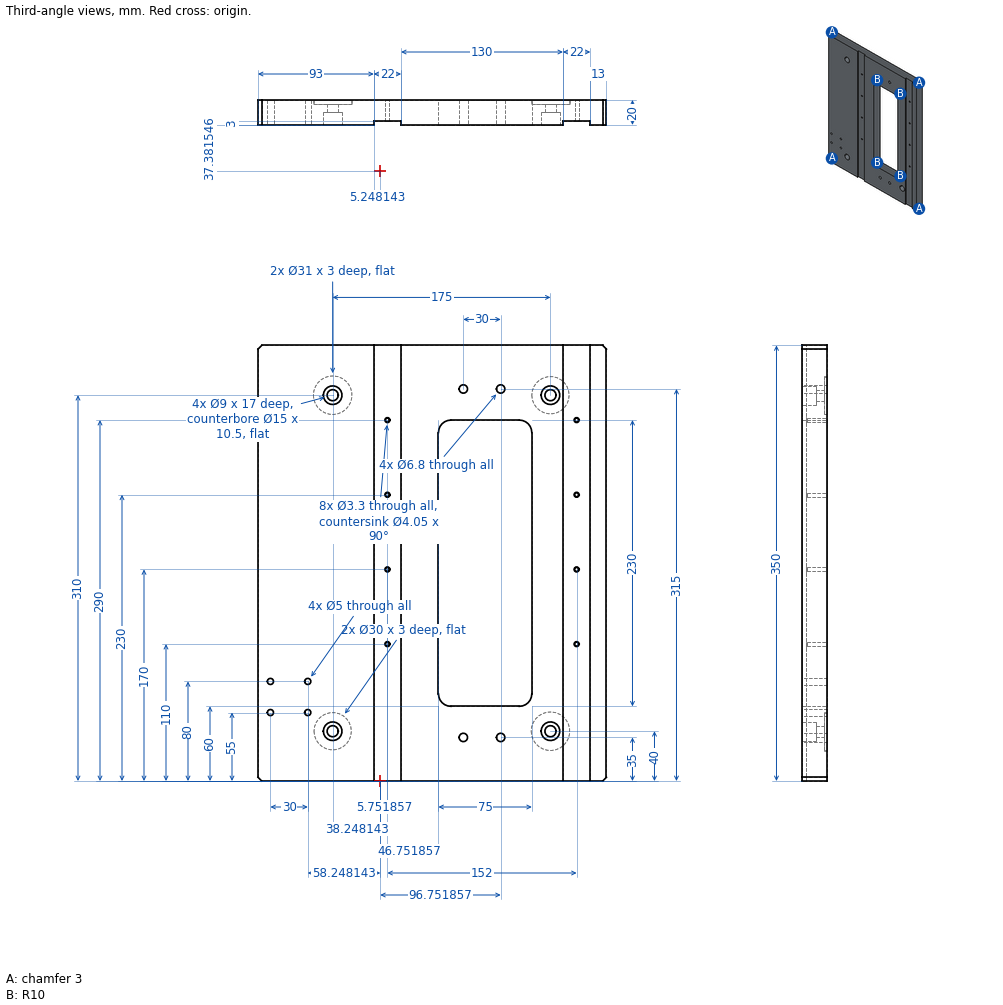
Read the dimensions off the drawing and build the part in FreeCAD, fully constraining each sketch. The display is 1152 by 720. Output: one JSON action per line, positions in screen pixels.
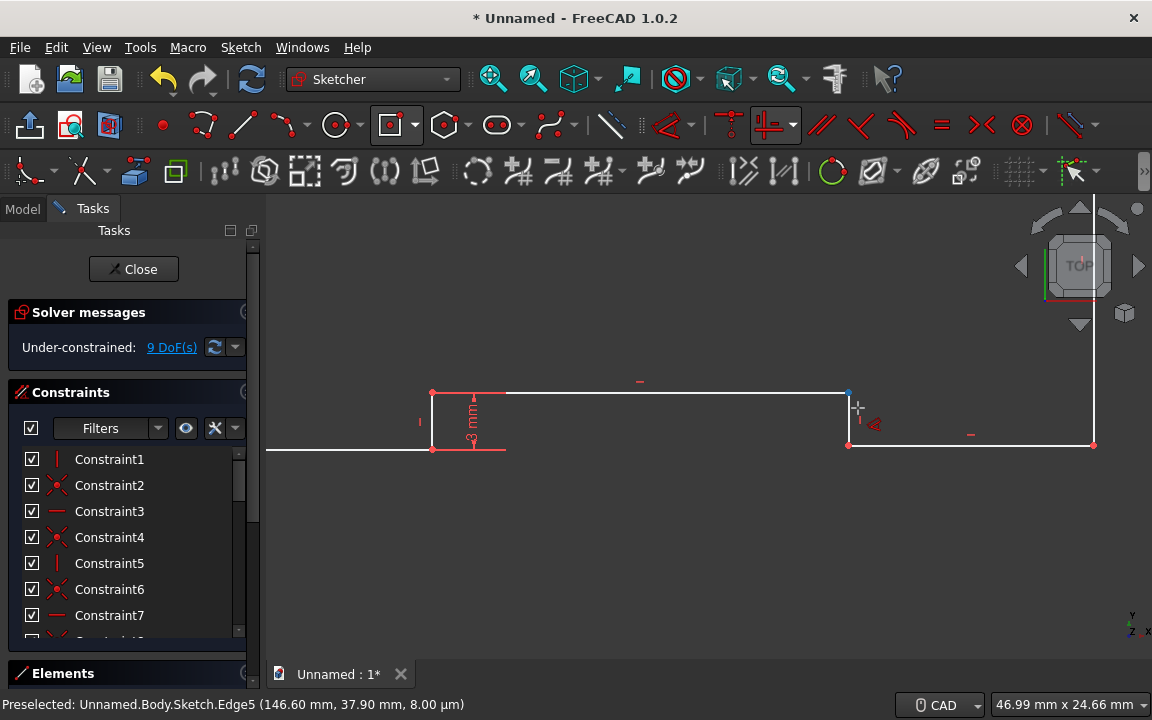
{"action": "left_click", "coordinate": [849, 409]}
{"action": "left_click", "coordinate": [883, 419]}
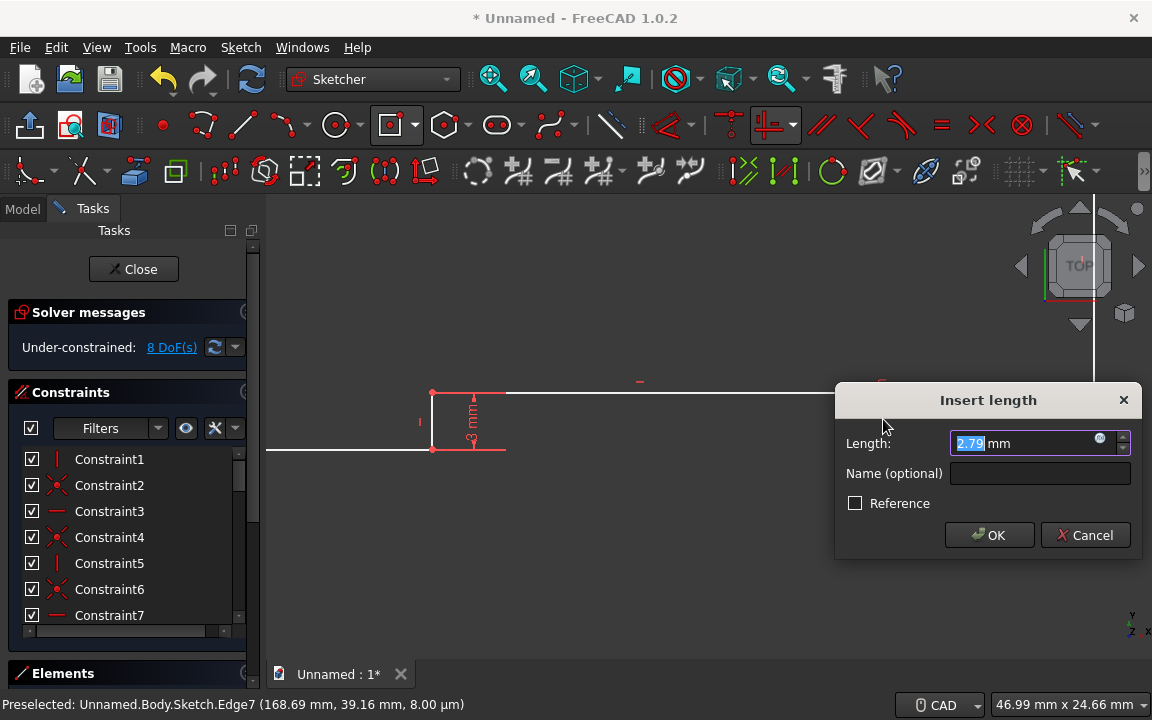
{"action": "type", "text": "3"}
{"action": "key", "text": "Return"}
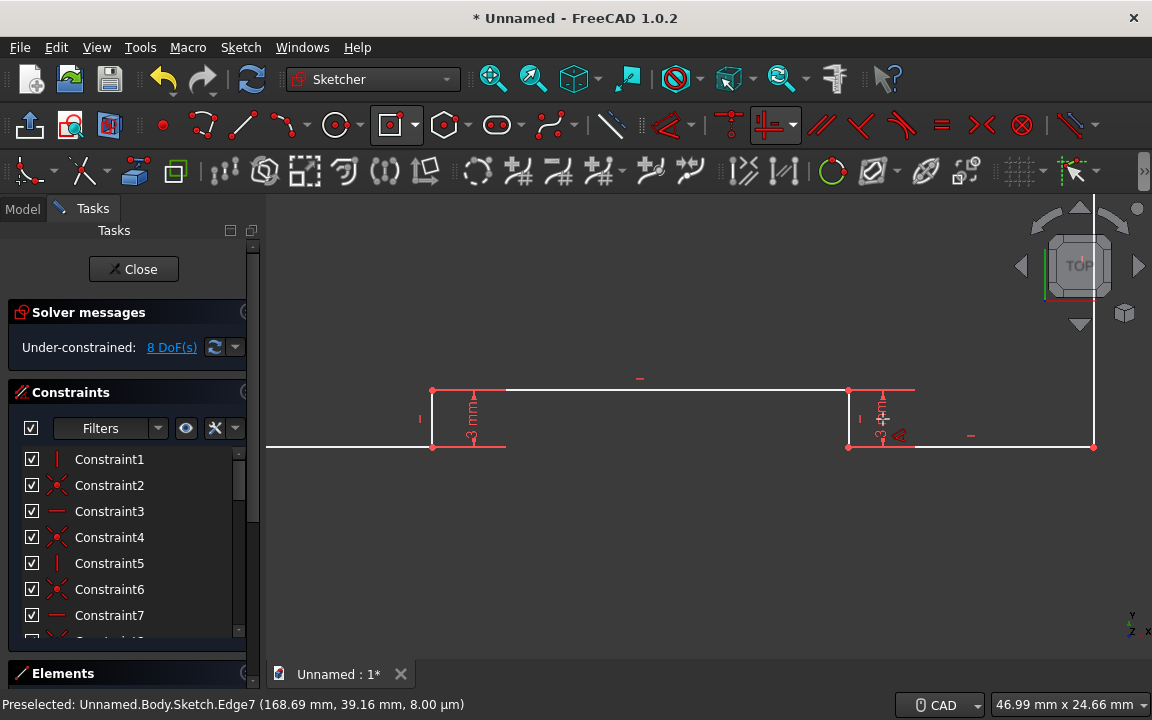
{"action": "scroll", "coordinate": [859, 408], "scroll_direction": "down", "scroll_amount": 12}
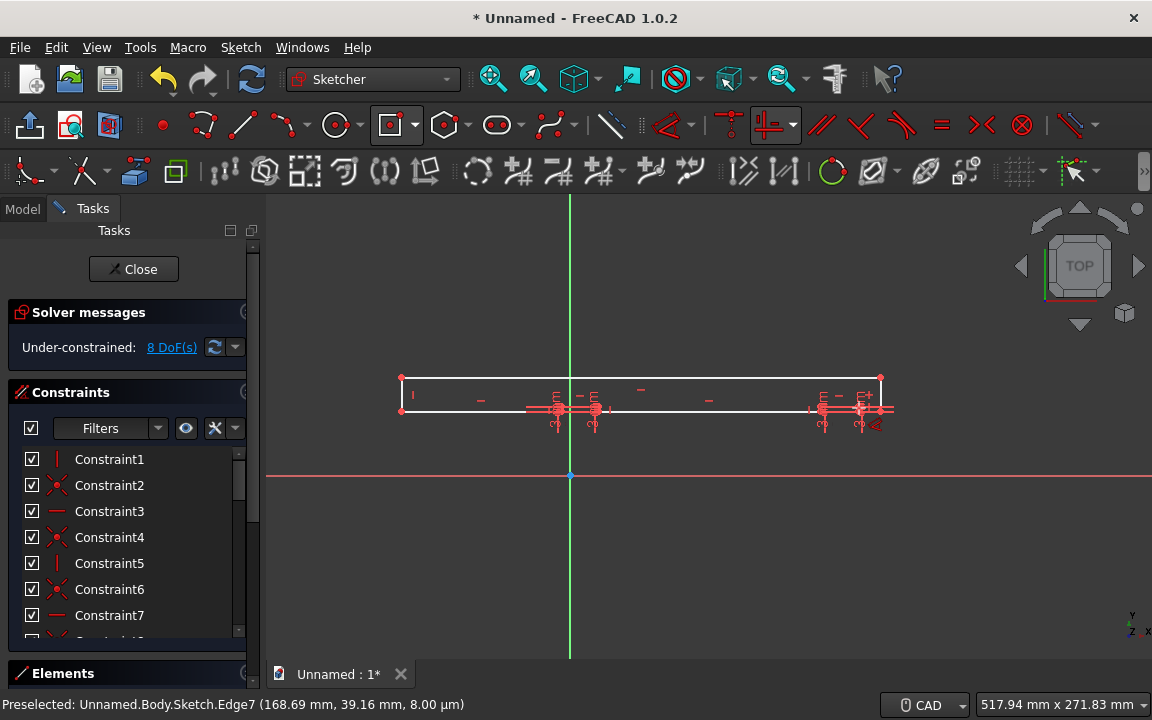
{"action": "scroll", "coordinate": [573, 407], "scroll_direction": "up", "scroll_amount": 9}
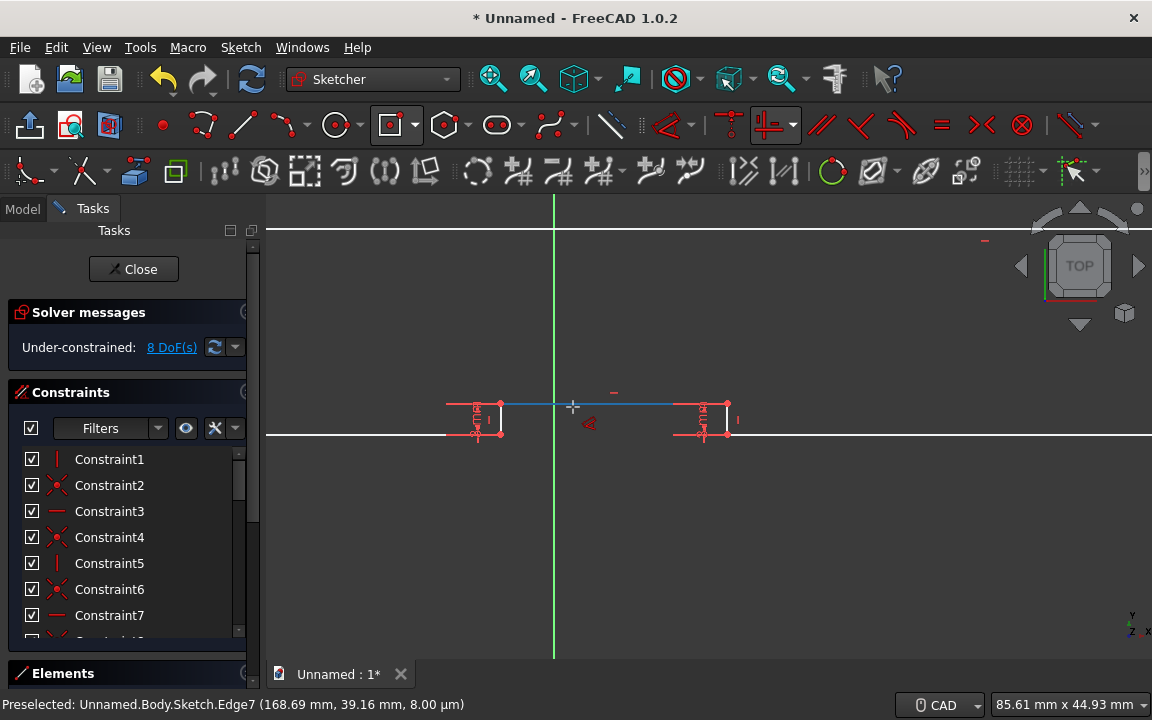
{"action": "left_click", "coordinate": [569, 404]}
{"action": "left_click", "coordinate": [614, 370]}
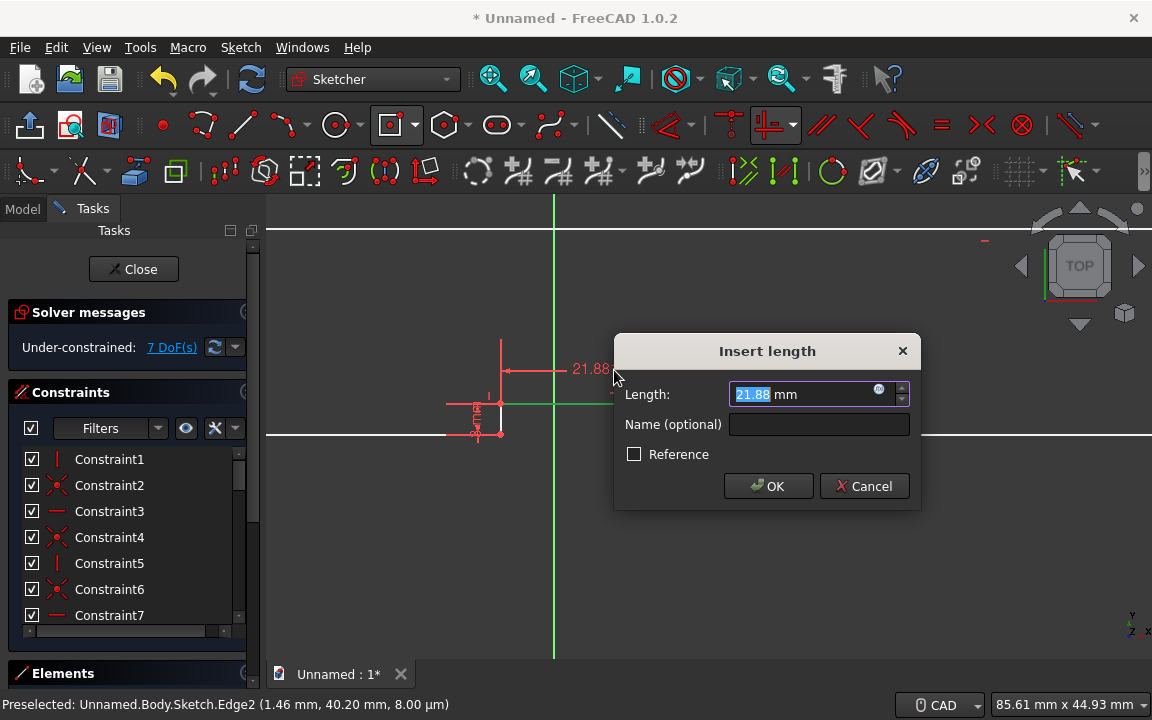
{"action": "type", "text": "22"}
{"action": "key", "text": "Return"}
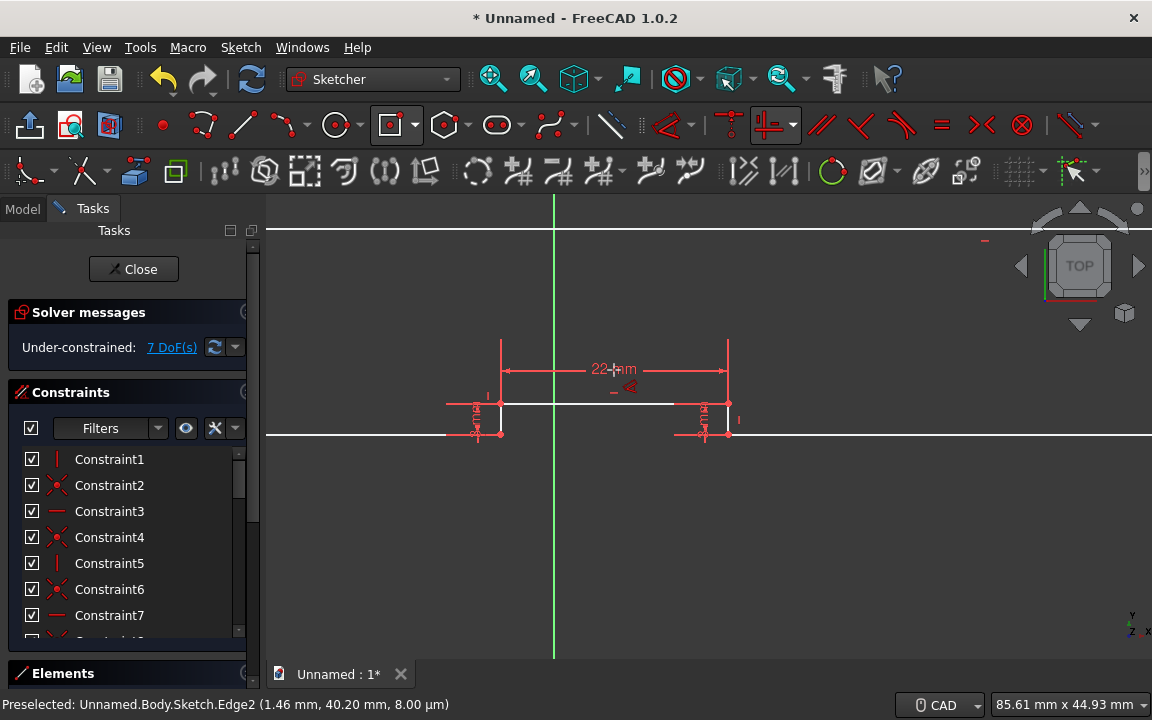
{"action": "scroll", "coordinate": [572, 407], "scroll_direction": "down", "scroll_amount": 9}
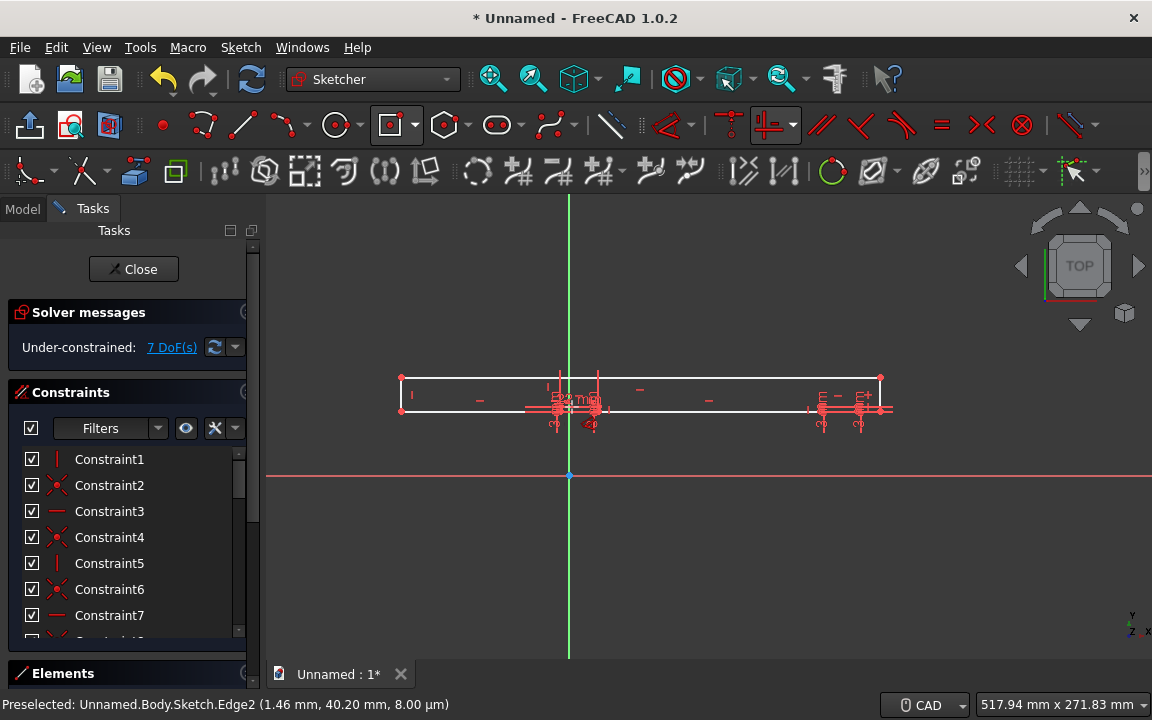
{"action": "left_click", "coordinate": [831, 407]}
{"action": "left_click", "coordinate": [839, 441]}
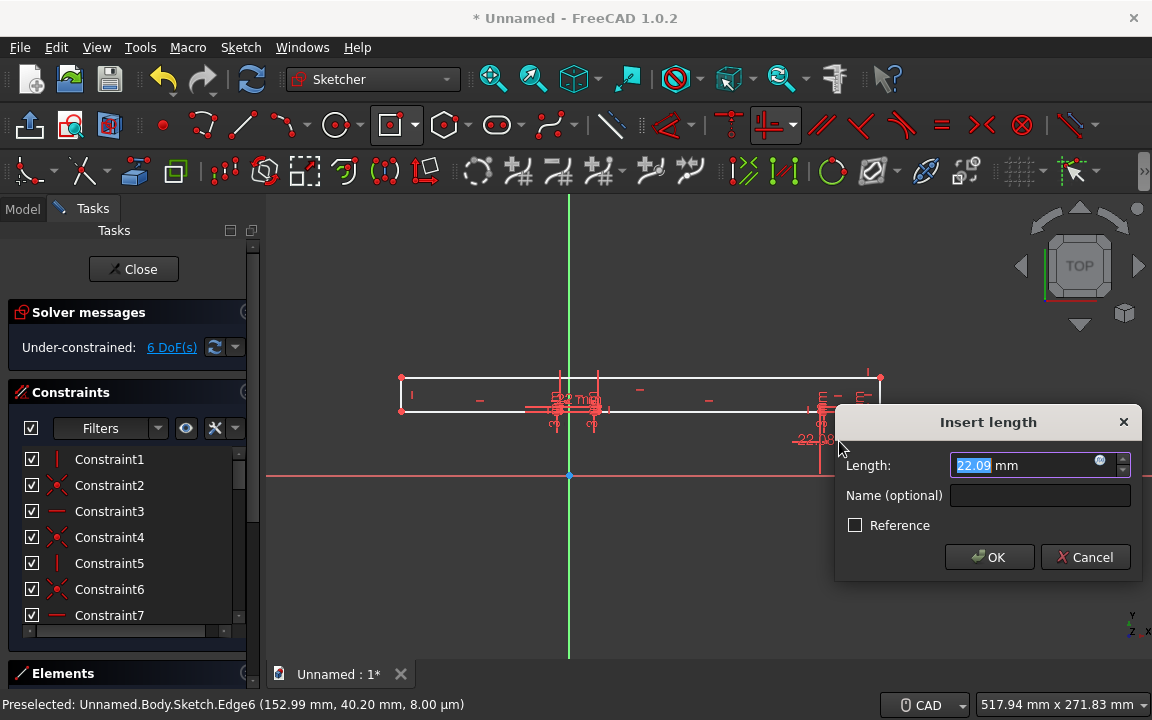
{"action": "type", "text": "22"}
{"action": "key", "text": "Return"}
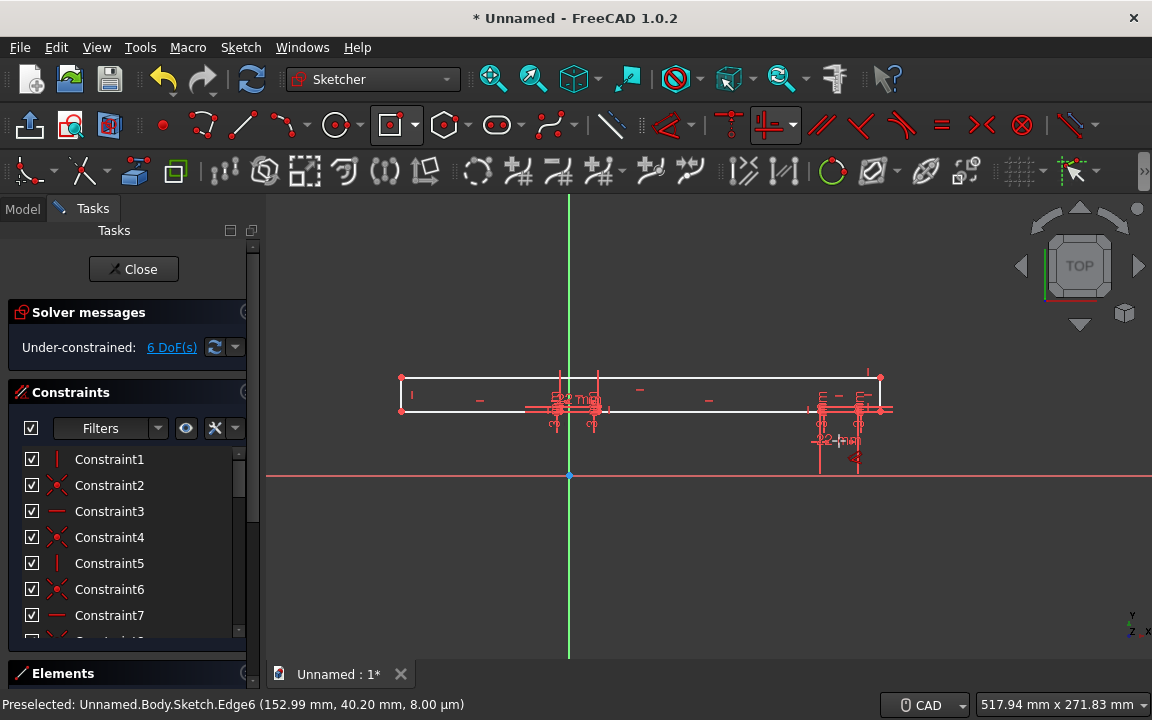
{"action": "scroll", "coordinate": [869, 412], "scroll_direction": "up", "scroll_amount": 3}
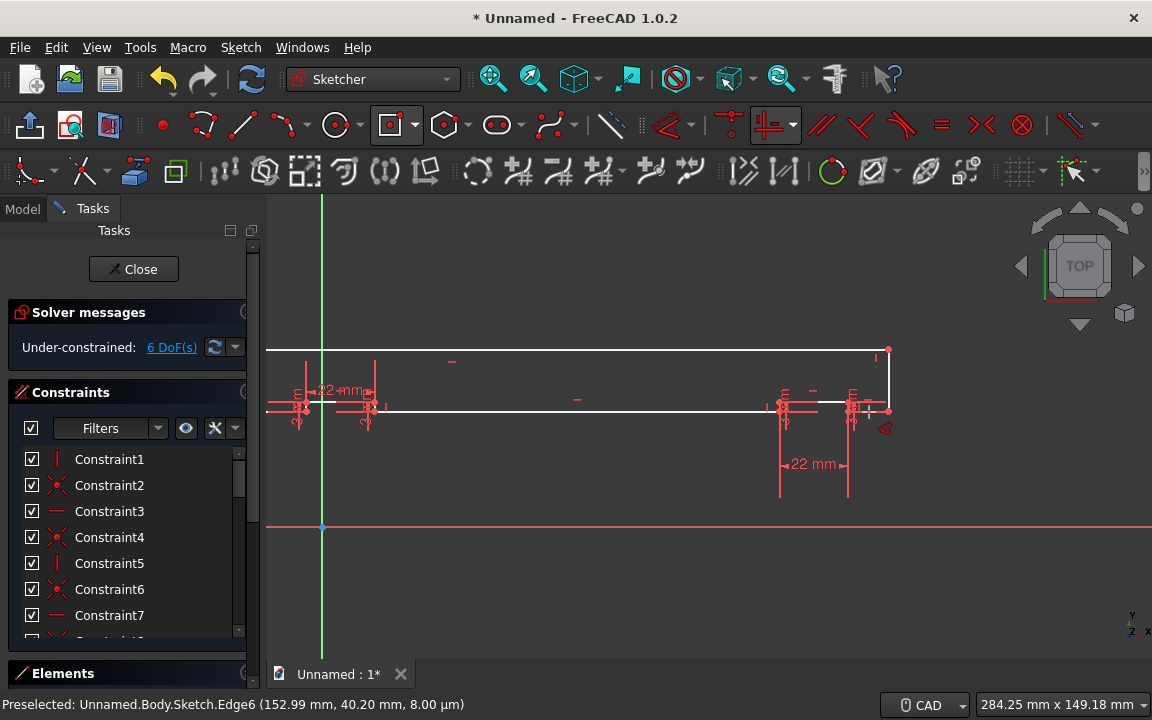
{"action": "left_click", "coordinate": [868, 412]}
{"action": "left_click", "coordinate": [868, 378]}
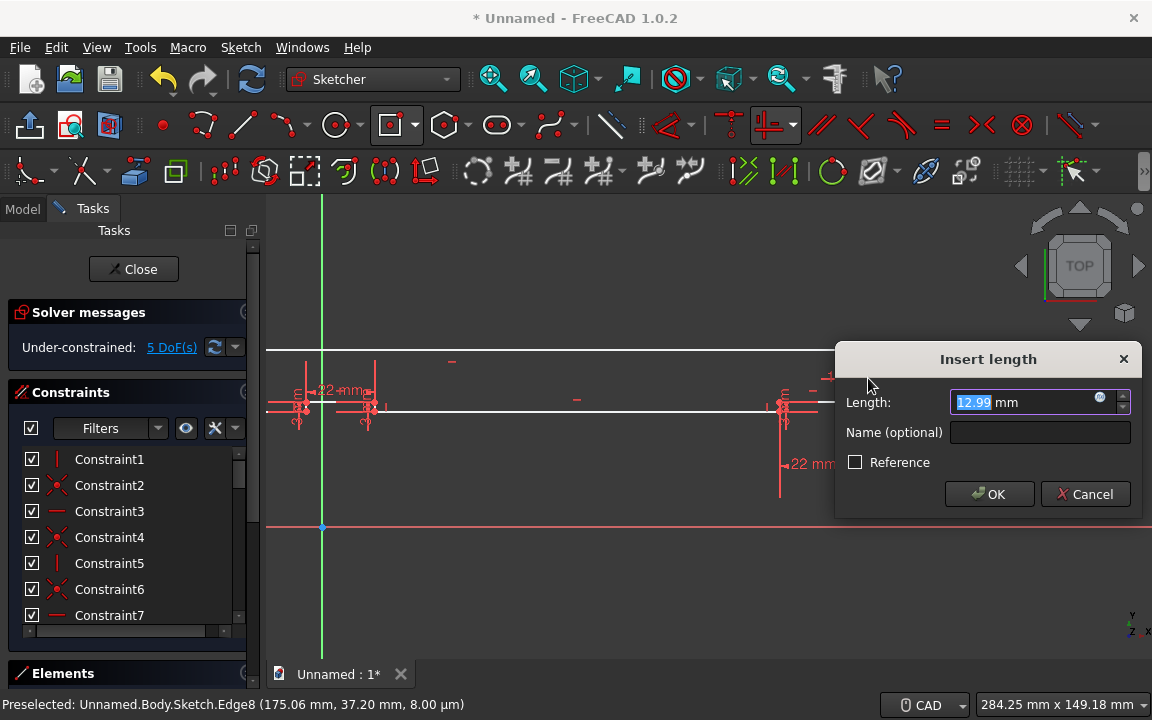
{"action": "type", "text": "13"}
{"action": "key", "text": "Return"}